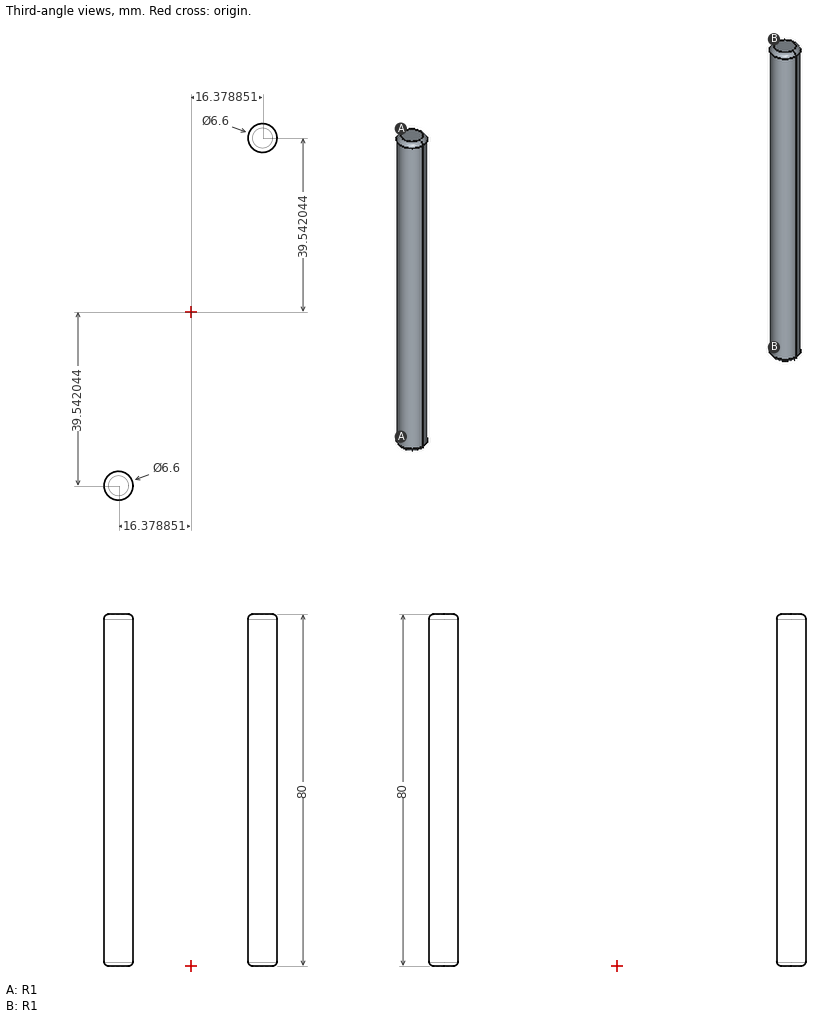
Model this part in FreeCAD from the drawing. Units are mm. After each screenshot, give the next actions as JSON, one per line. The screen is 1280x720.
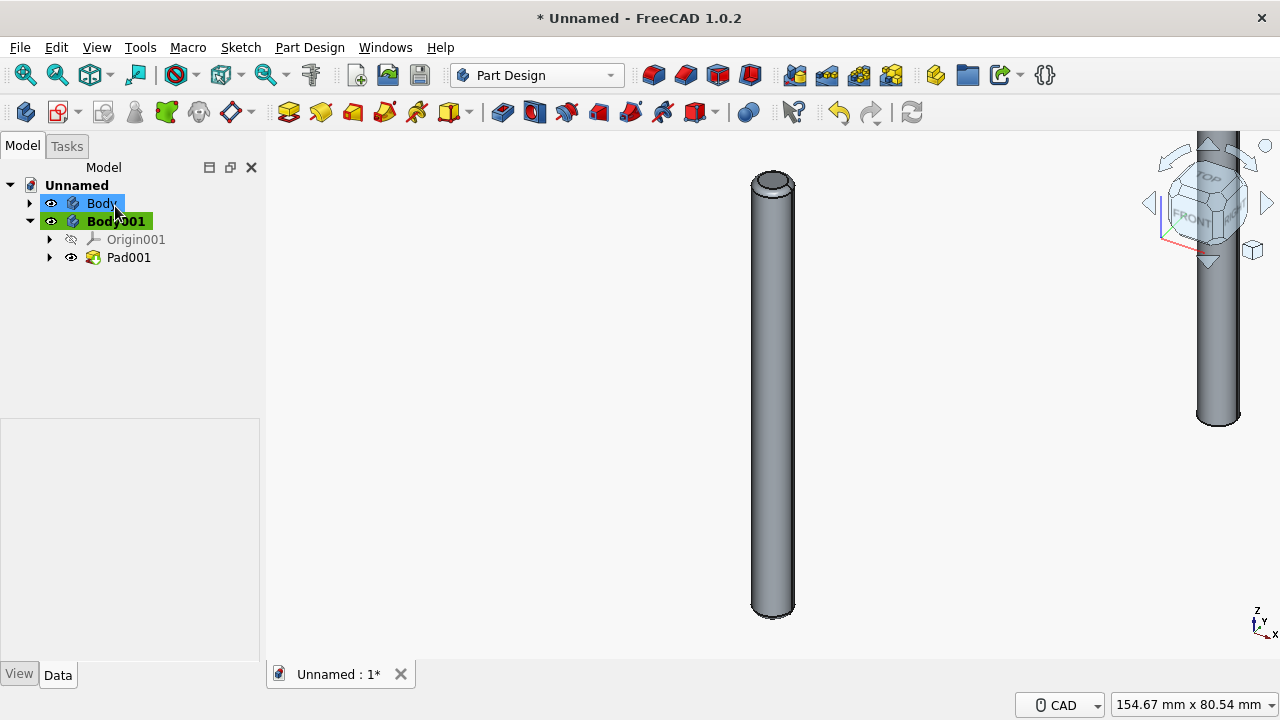
{"action": "left_click", "coordinate": [26, 76]}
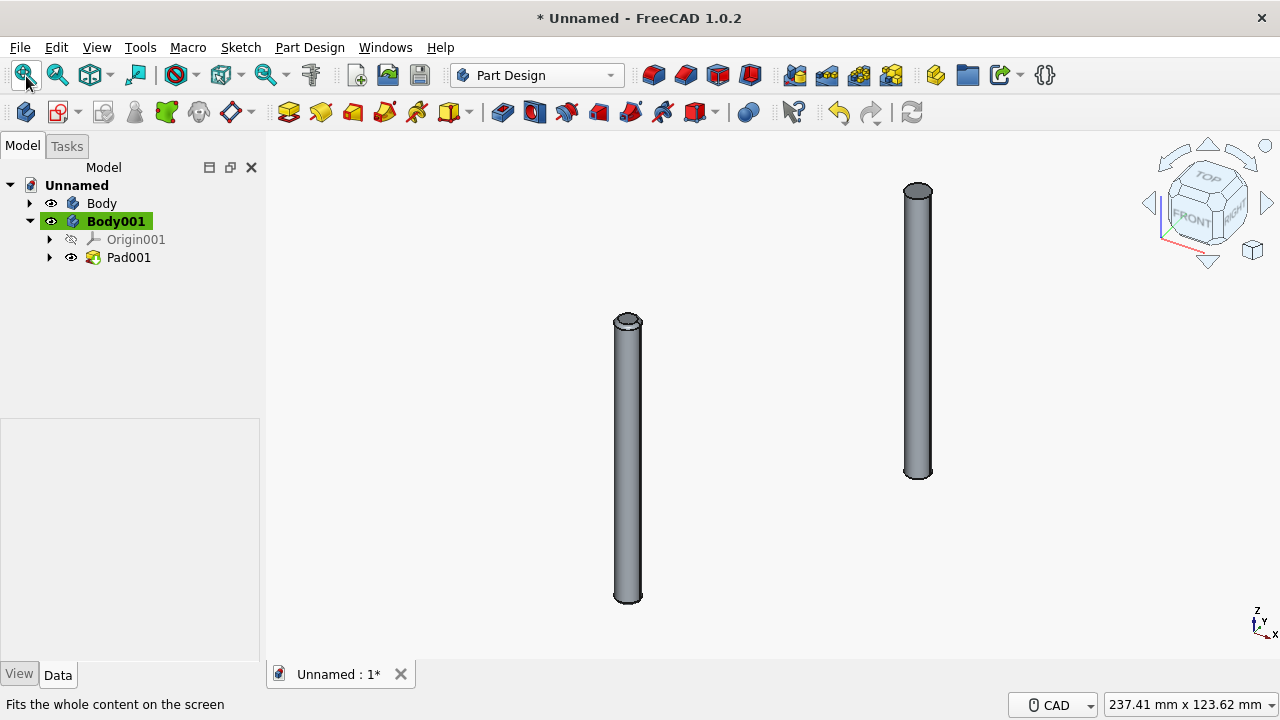
{"action": "left_click", "coordinate": [908, 476]}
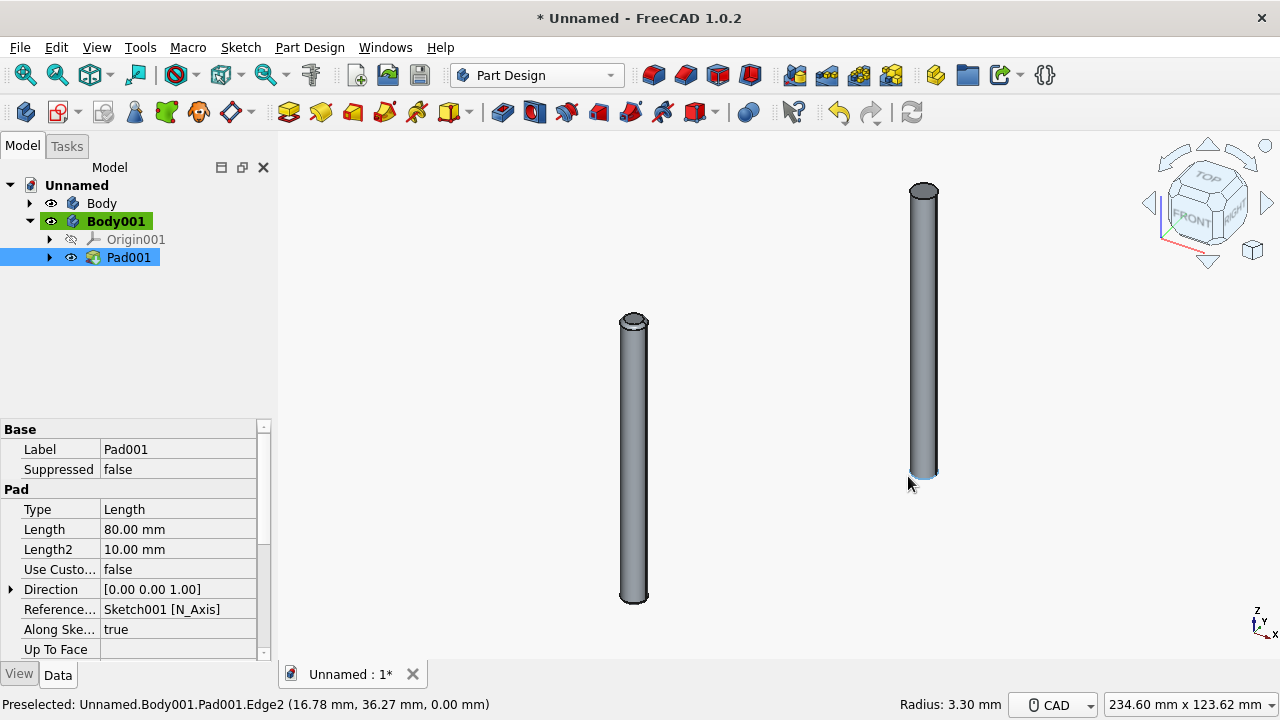
{"action": "left_click", "coordinate": [912, 186], "text": "ctrl"}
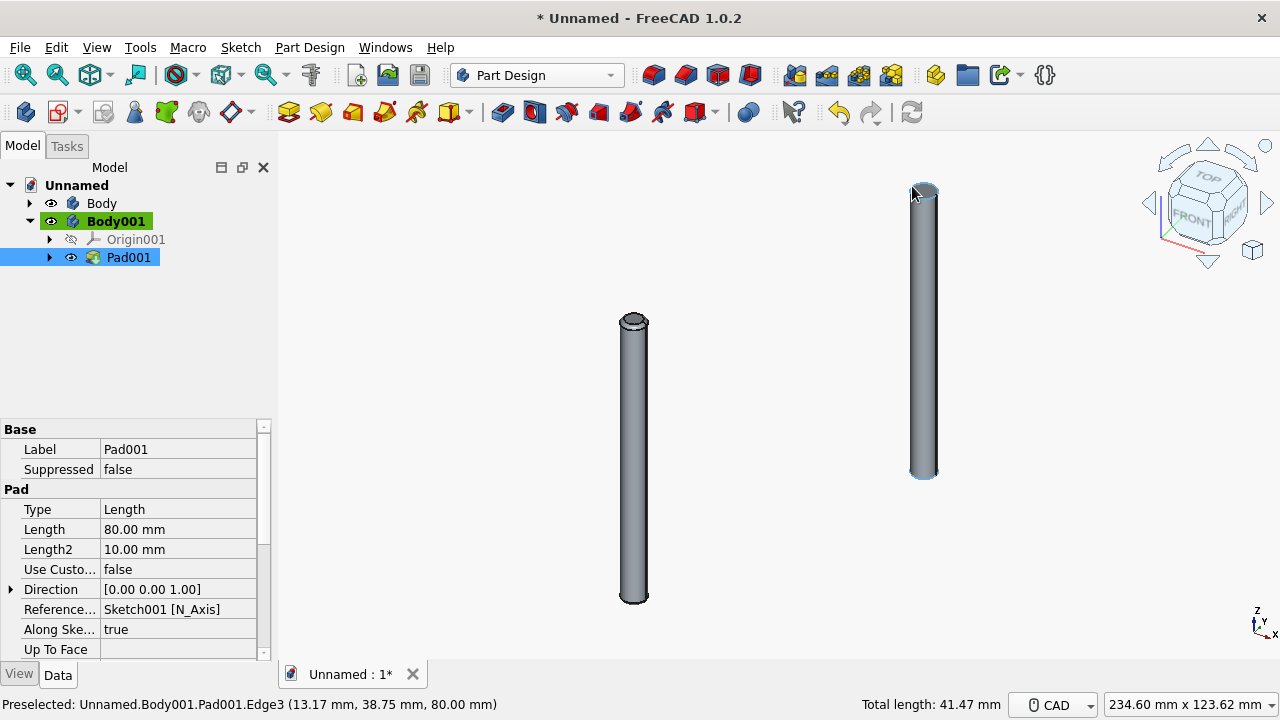
{"action": "left_click", "coordinate": [654, 76]}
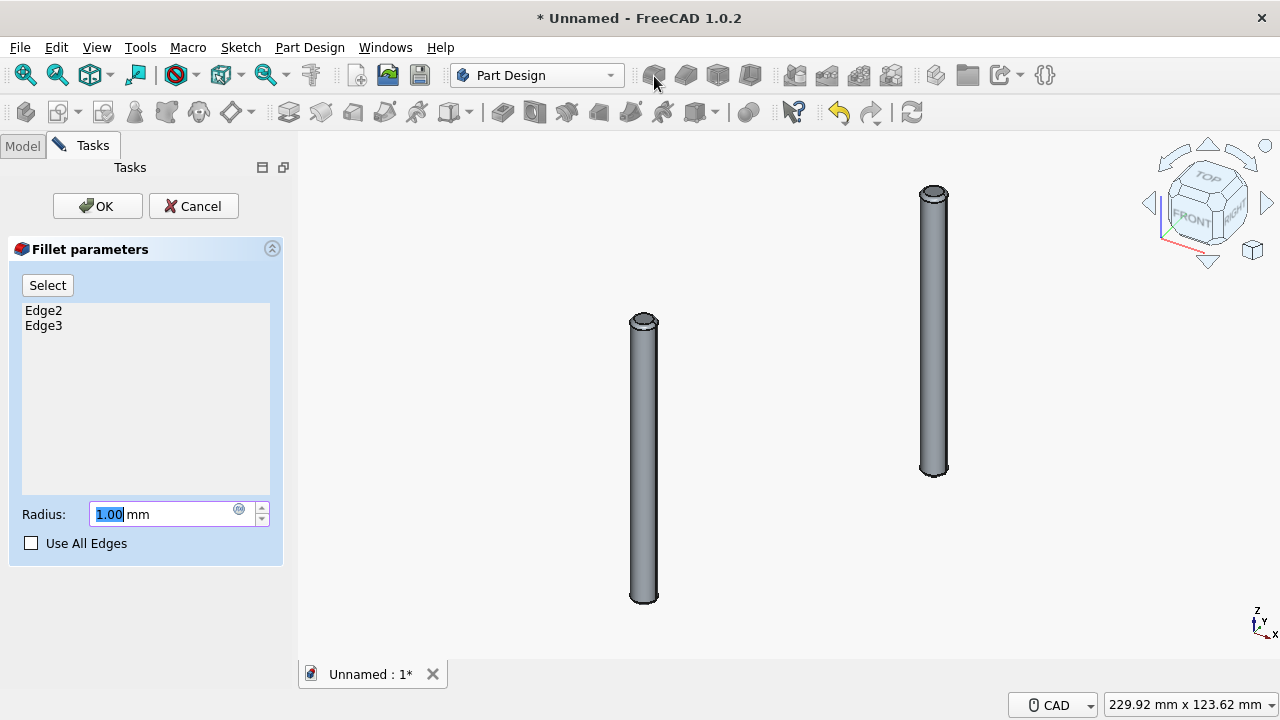
{"action": "type", "text": "1"}
{"action": "key", "text": "Tab"}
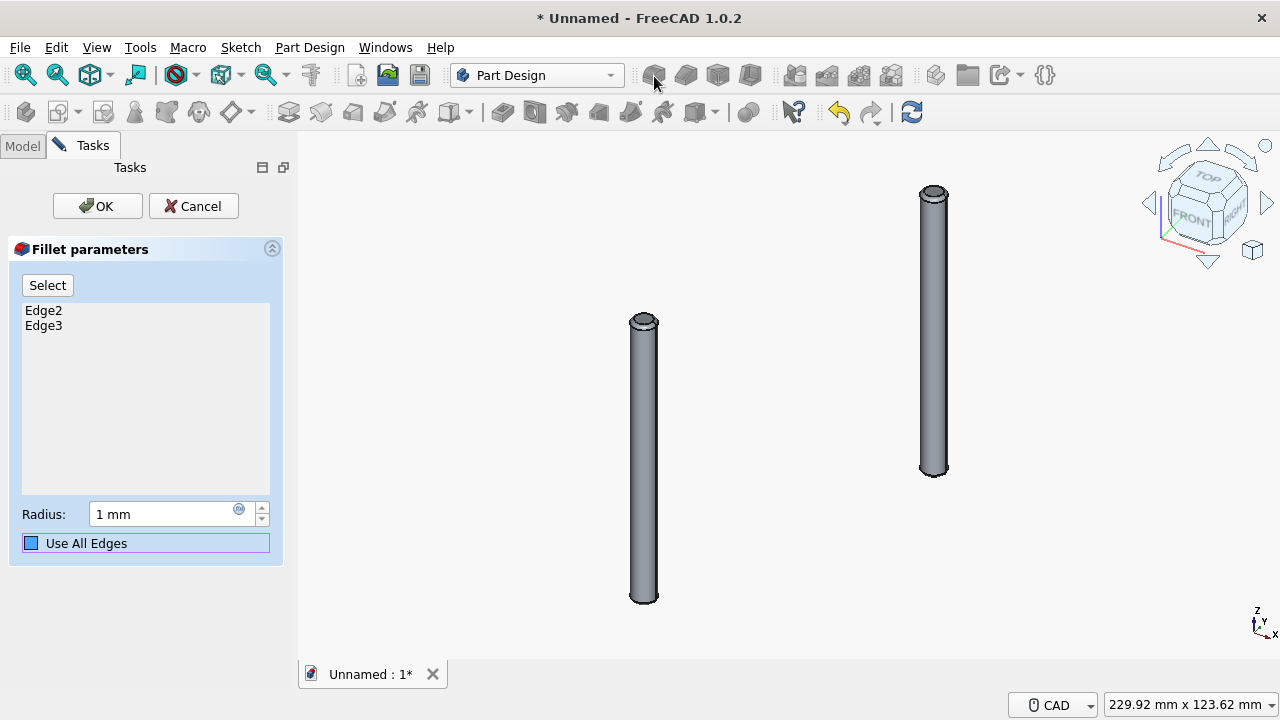
{"action": "left_click", "coordinate": [98, 206]}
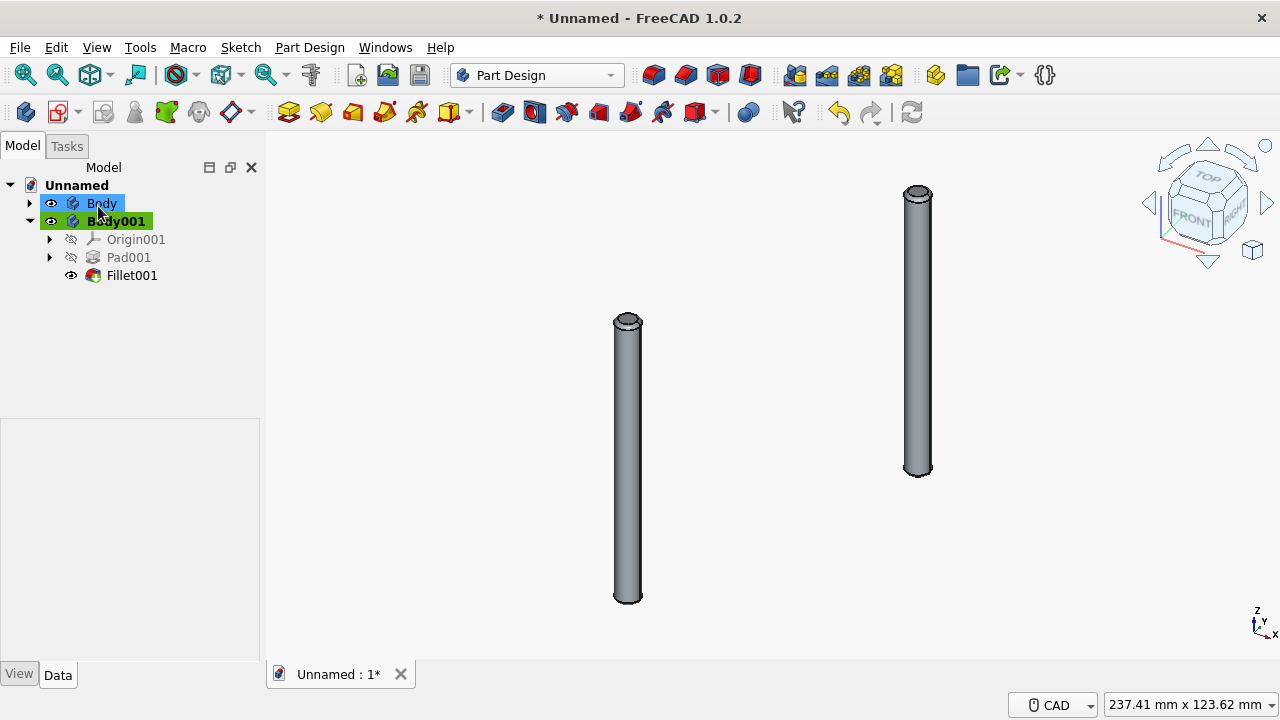
{"action": "key", "text": "0"}